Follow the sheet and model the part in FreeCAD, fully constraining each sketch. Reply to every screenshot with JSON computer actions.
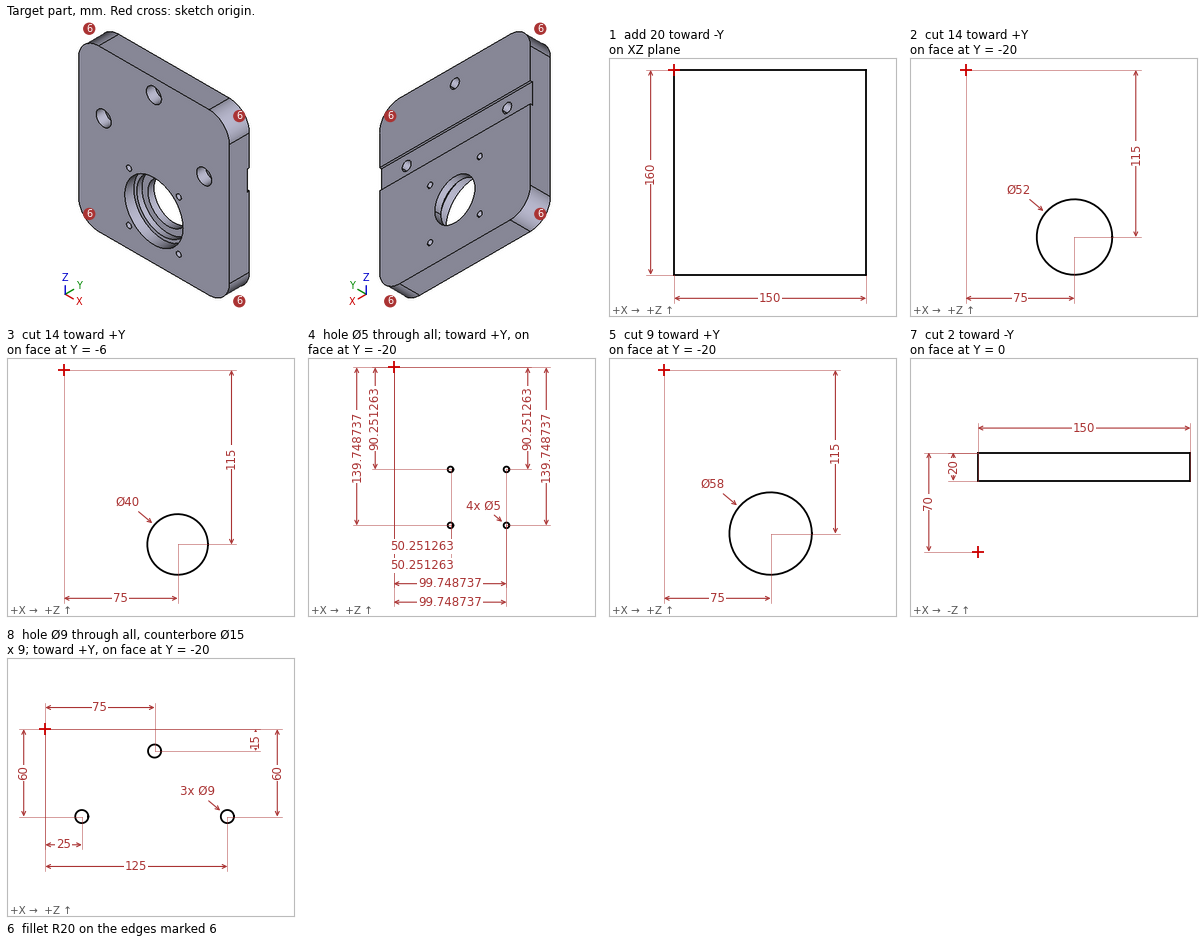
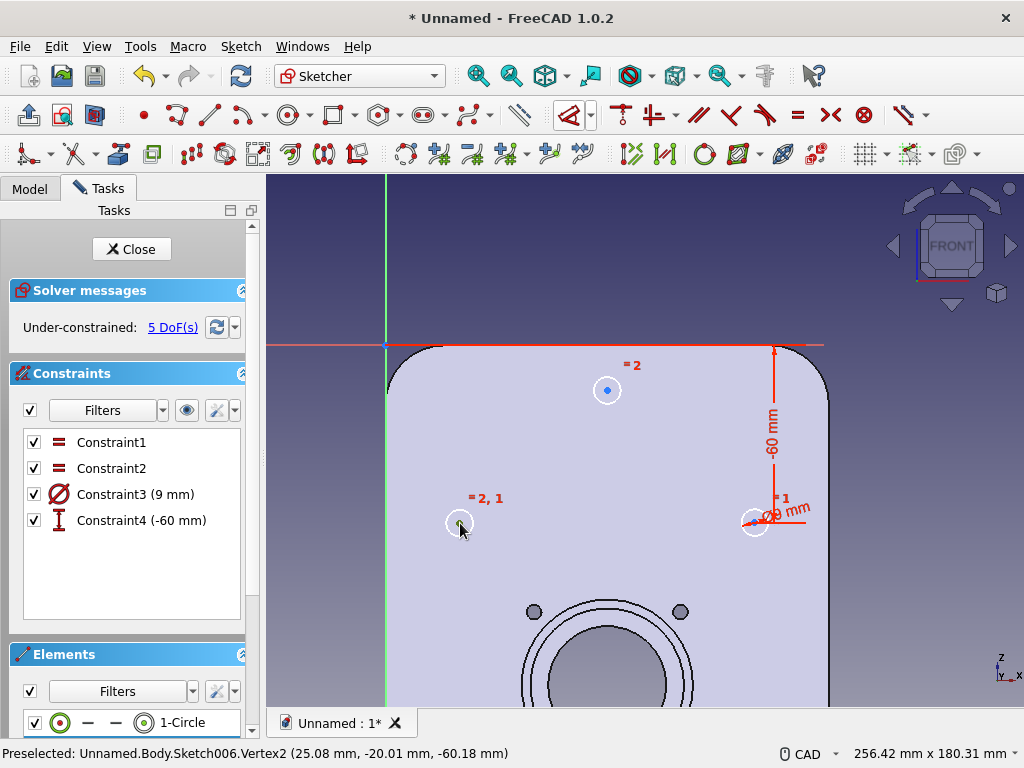
{"action": "key", "text": "l"}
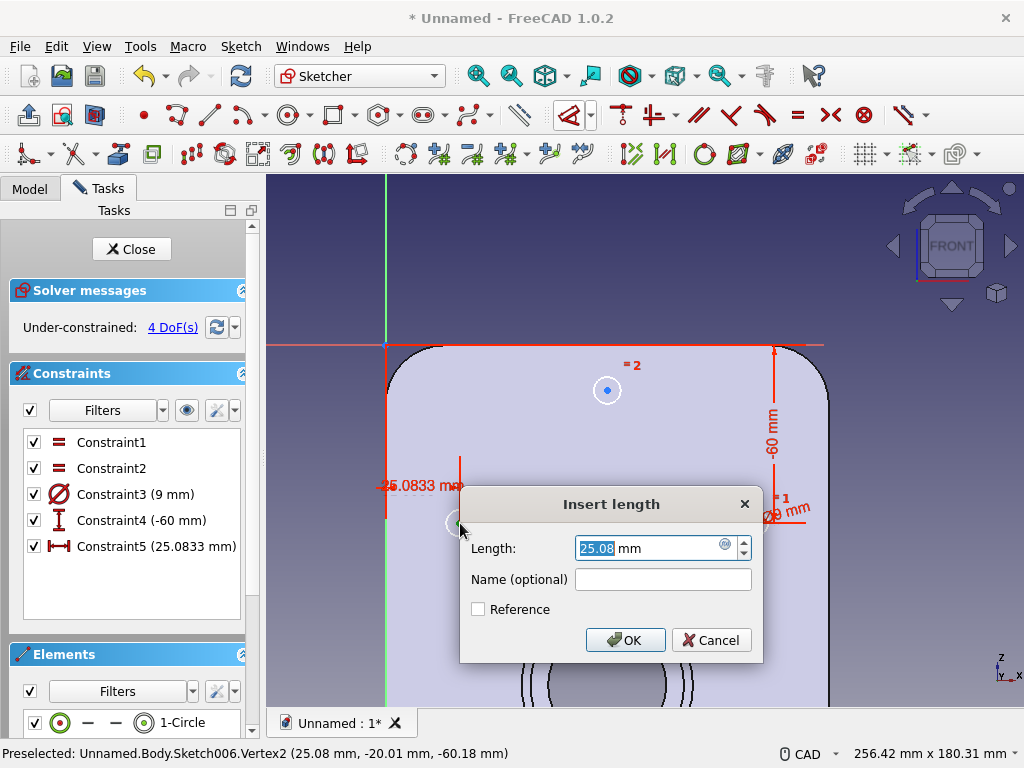
{"action": "type", "text": "25"}
{"action": "key", "text": "Return"}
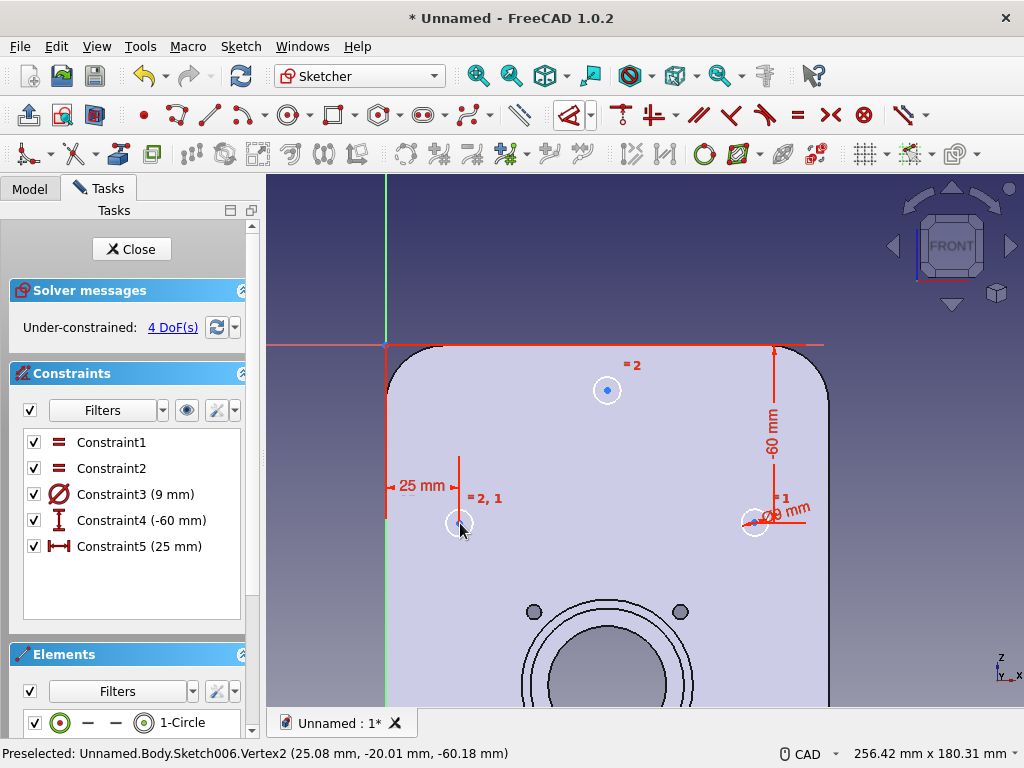
{"action": "left_click", "coordinate": [459, 523]}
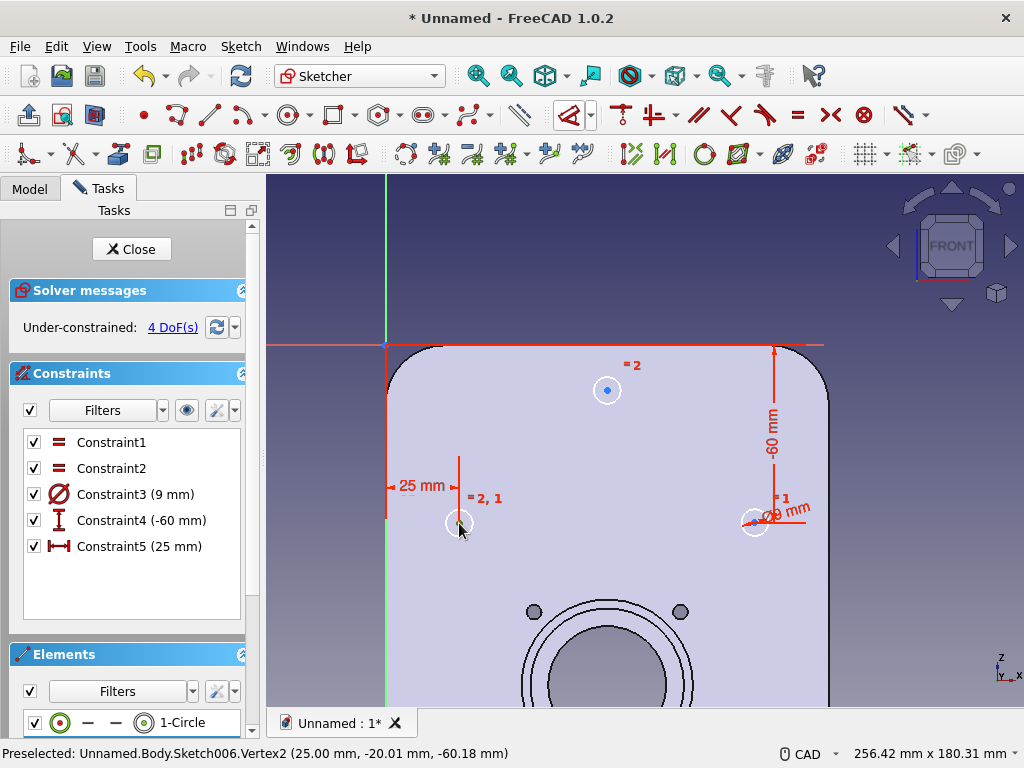
{"action": "key", "text": "i"}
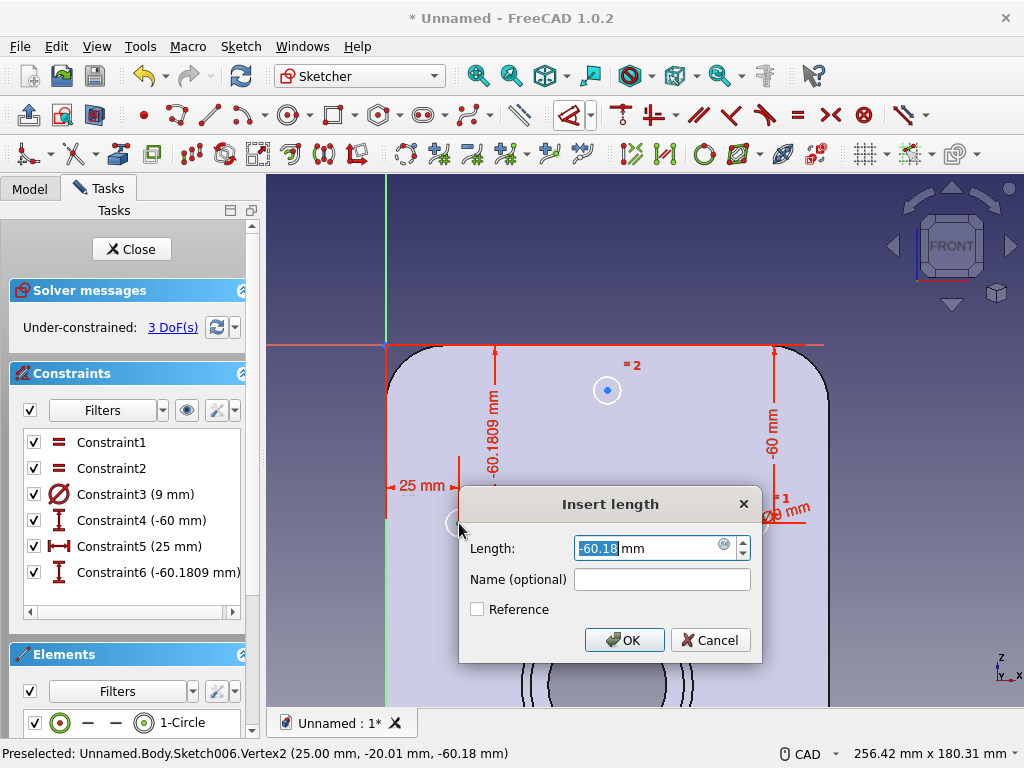
{"action": "type", "text": "-60"}
{"action": "key", "text": "Return"}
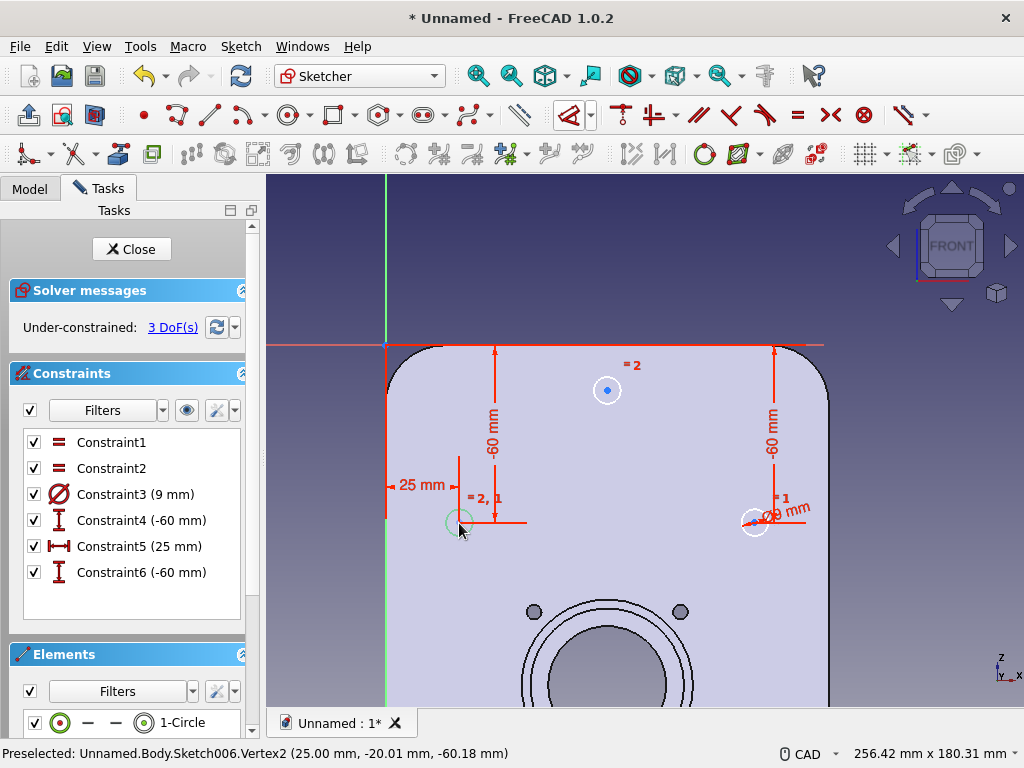
{"action": "left_click", "coordinate": [607, 390]}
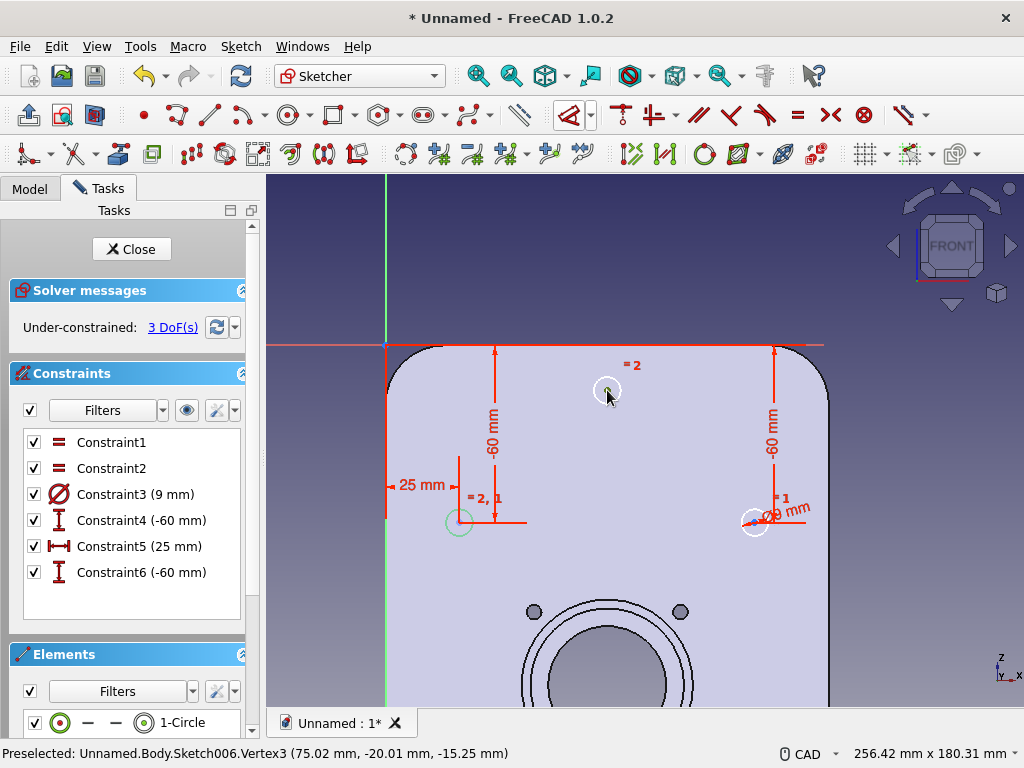
{"action": "key", "text": "l"}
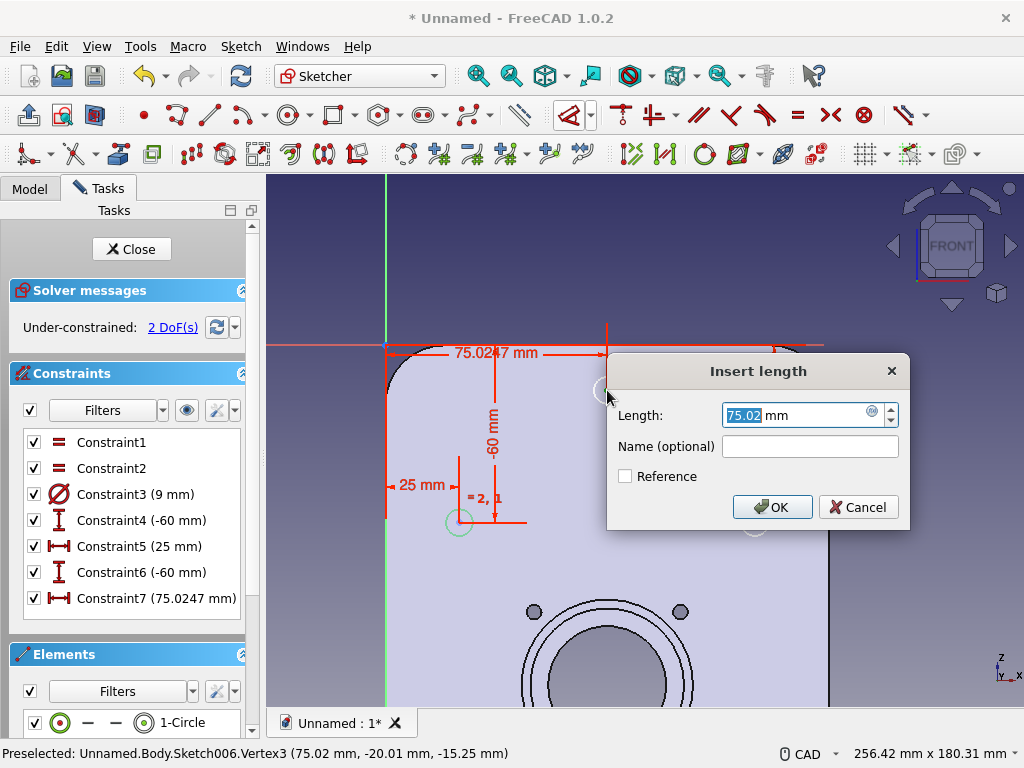
{"action": "type", "text": "75"}
{"action": "key", "text": "Return"}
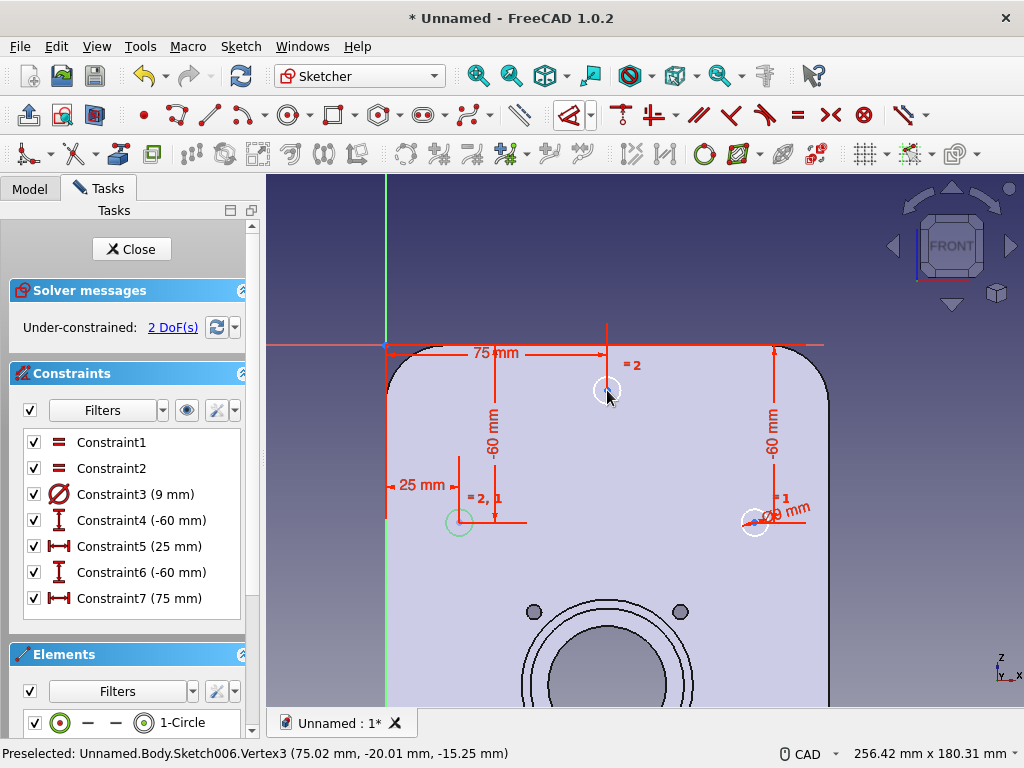
{"action": "left_click", "coordinate": [607, 390]}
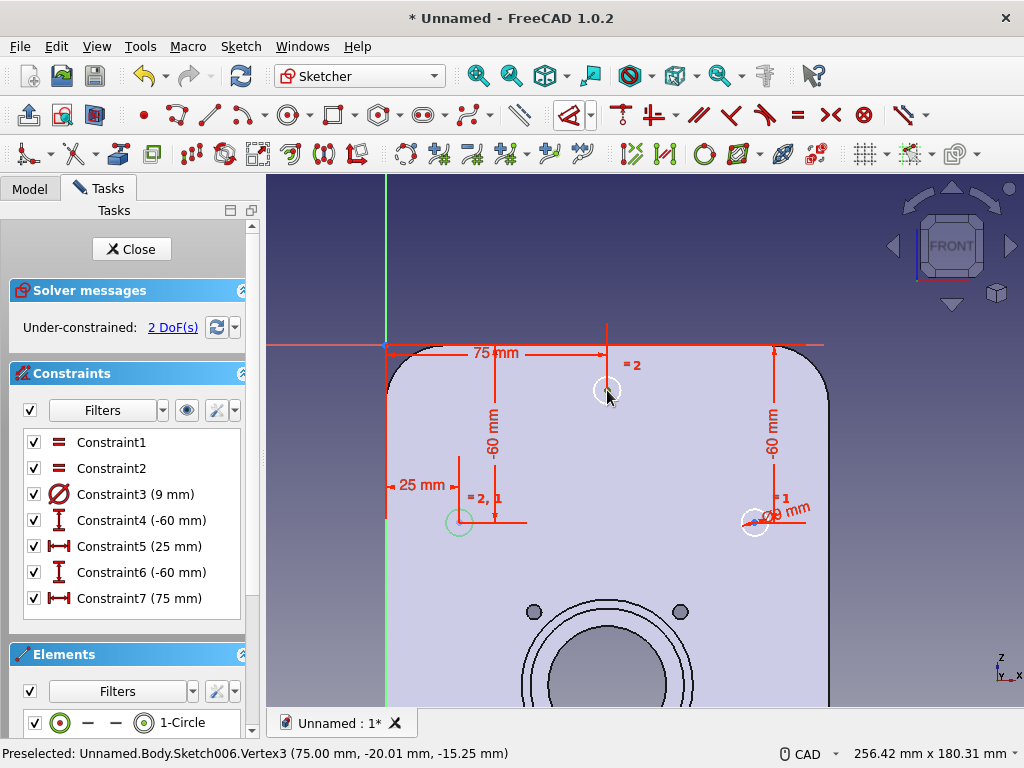
{"action": "key", "text": "i"}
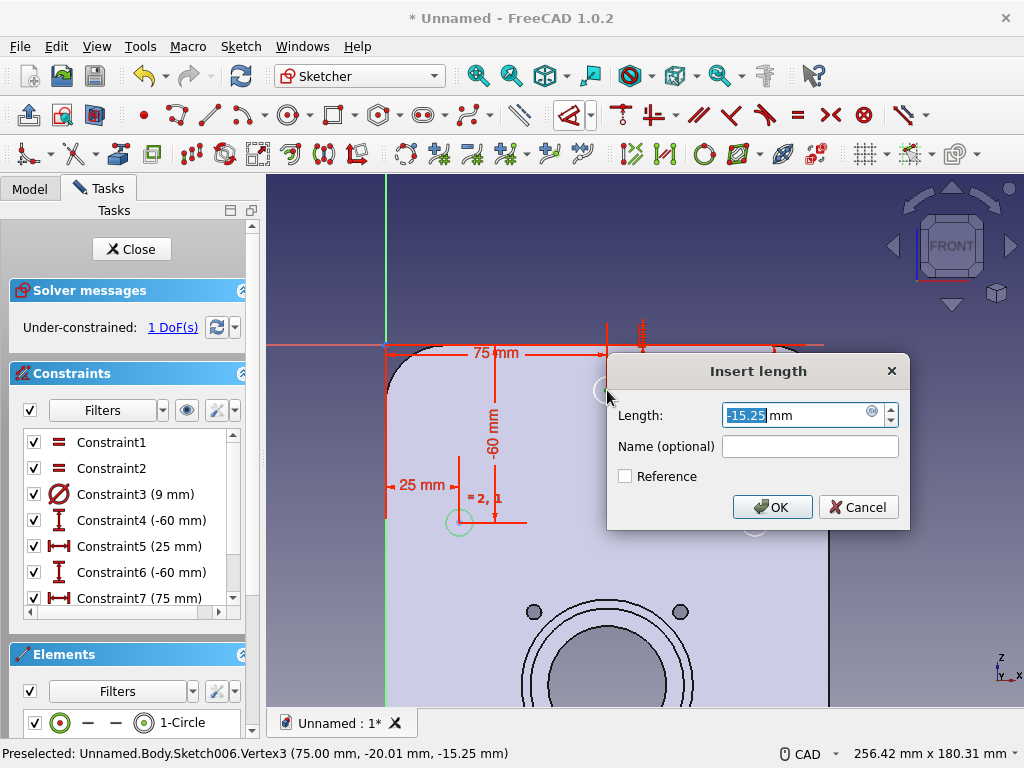
{"action": "type", "text": "-15"}
{"action": "key", "text": "Return"}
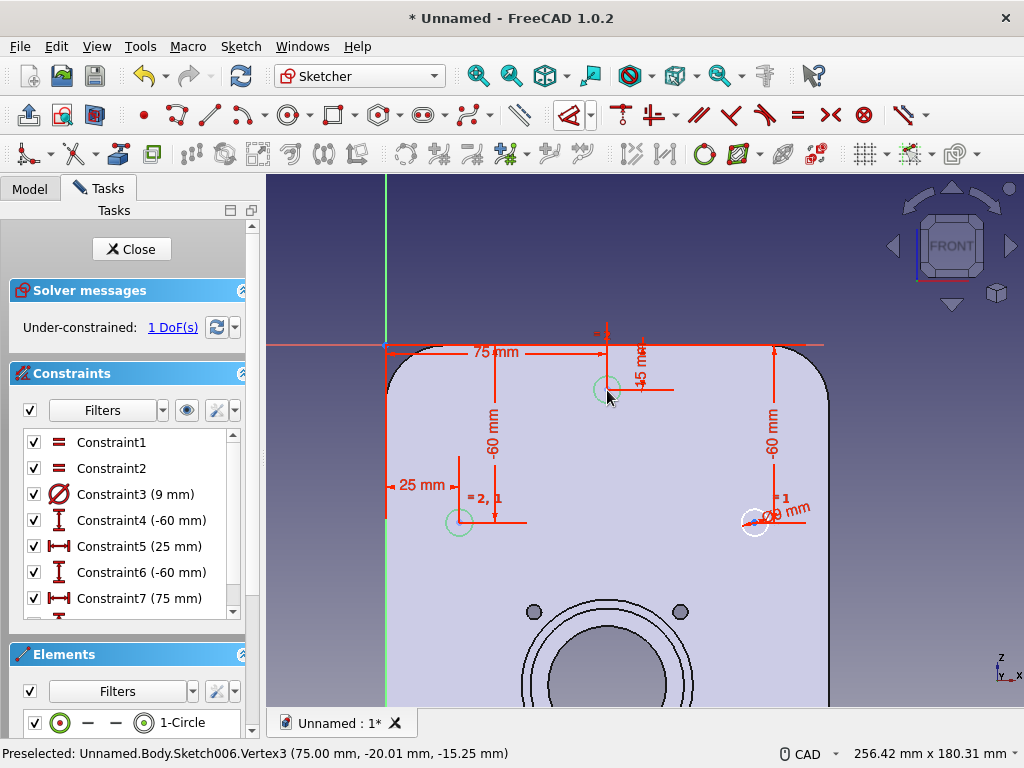
{"action": "left_click", "coordinate": [755, 523]}